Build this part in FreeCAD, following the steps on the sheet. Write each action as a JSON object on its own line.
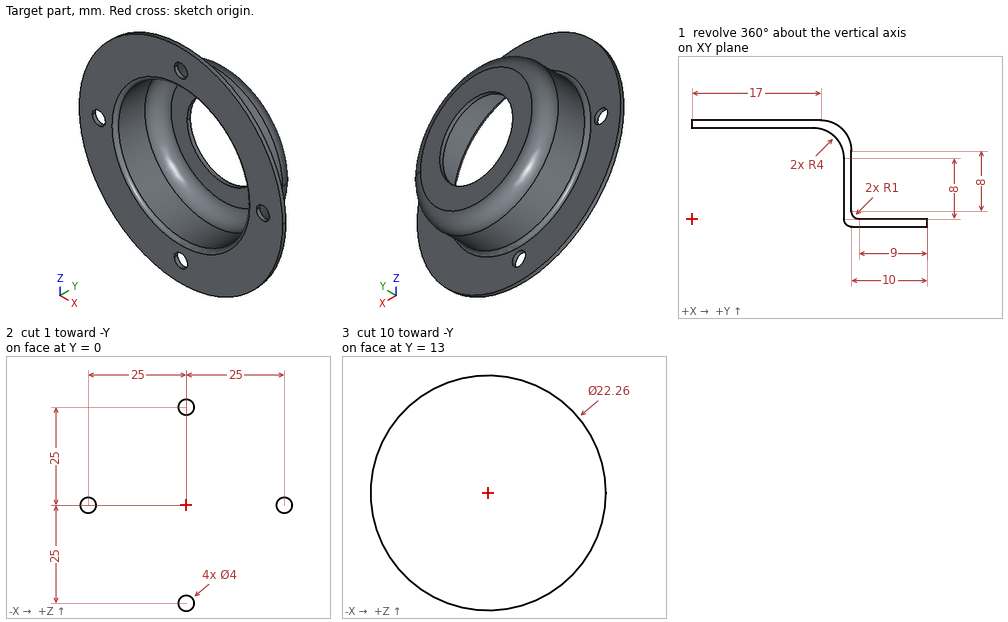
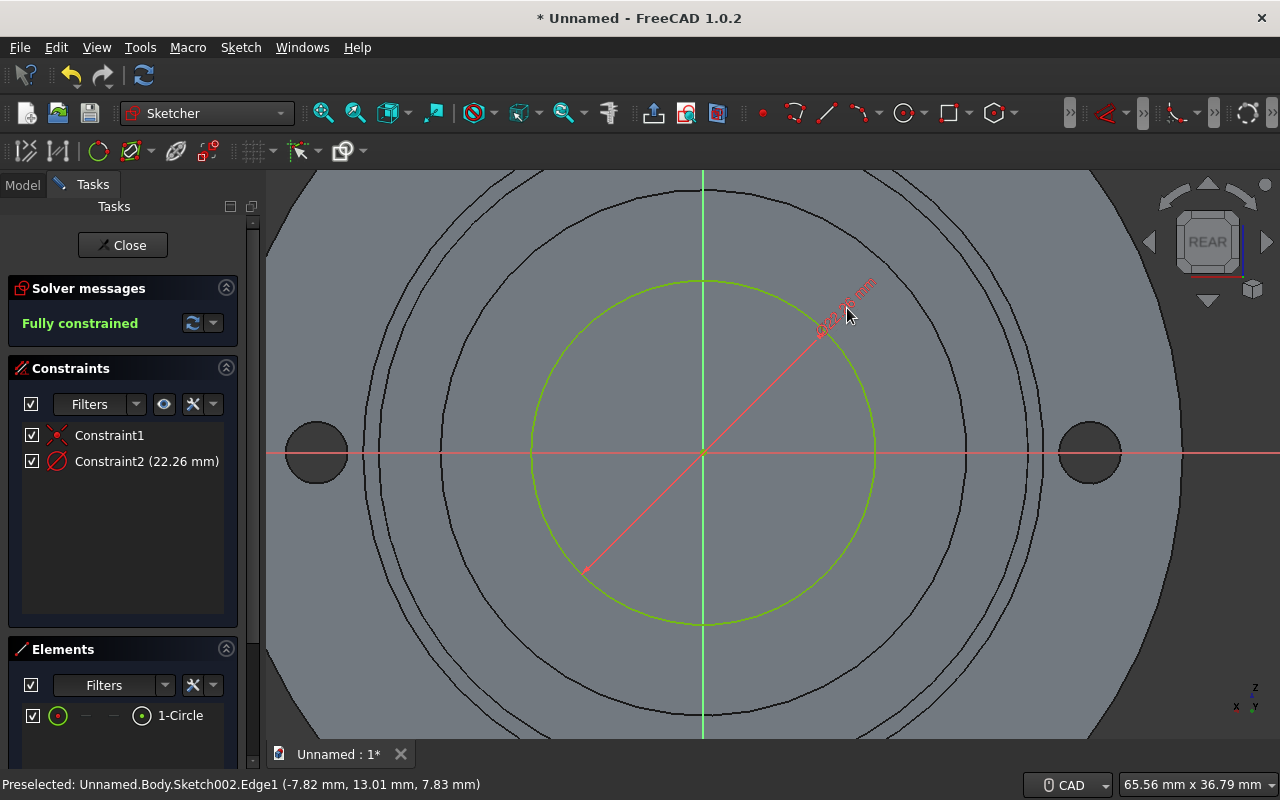
{"action": "left_click", "coordinate": [123, 245]}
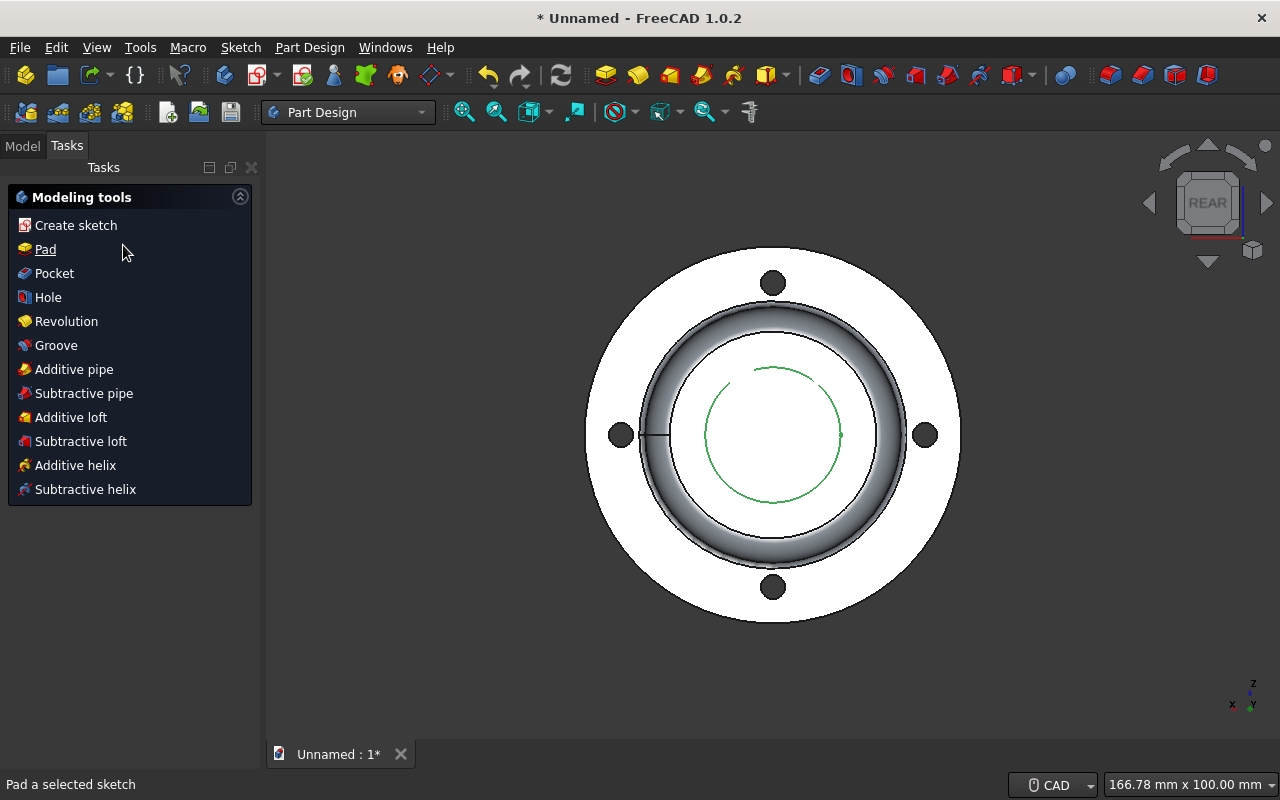
{"action": "left_click", "coordinate": [820, 76]}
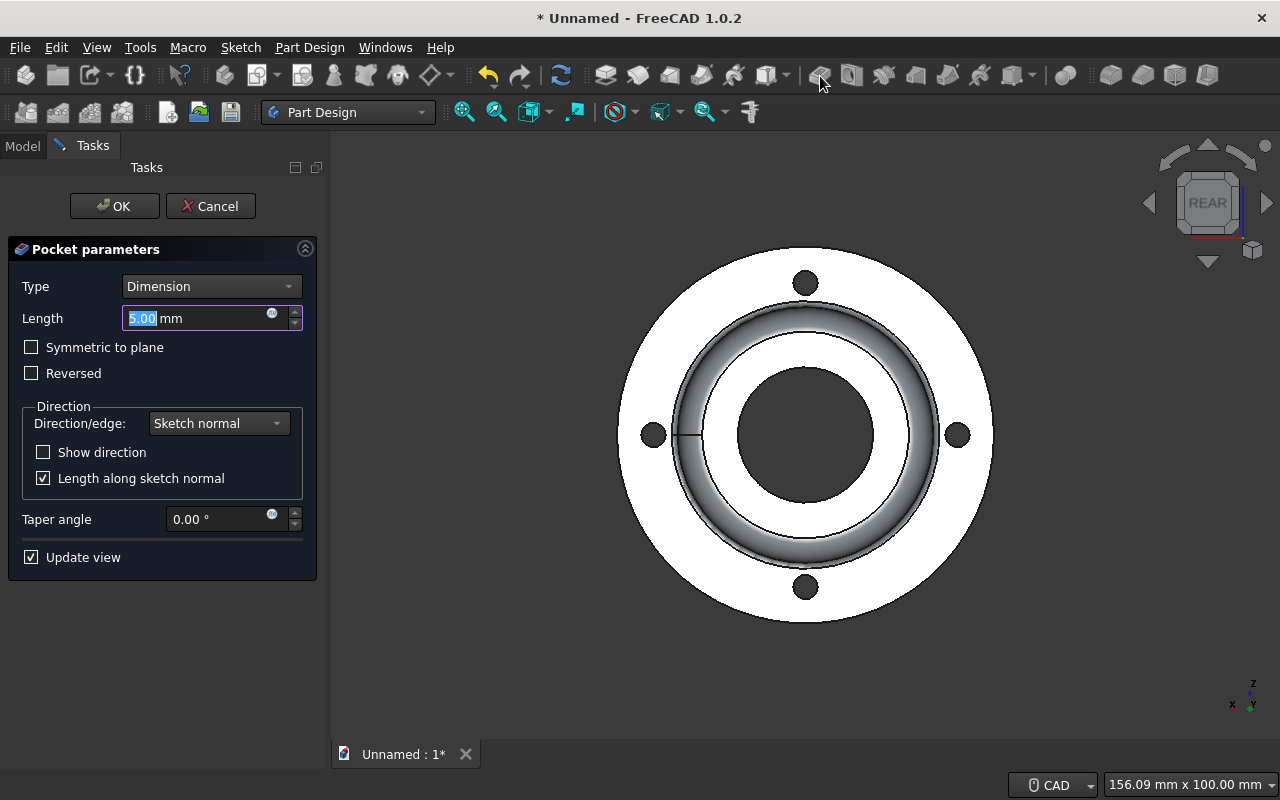
{"action": "type", "text": "10"}
{"action": "key", "text": "Tab"}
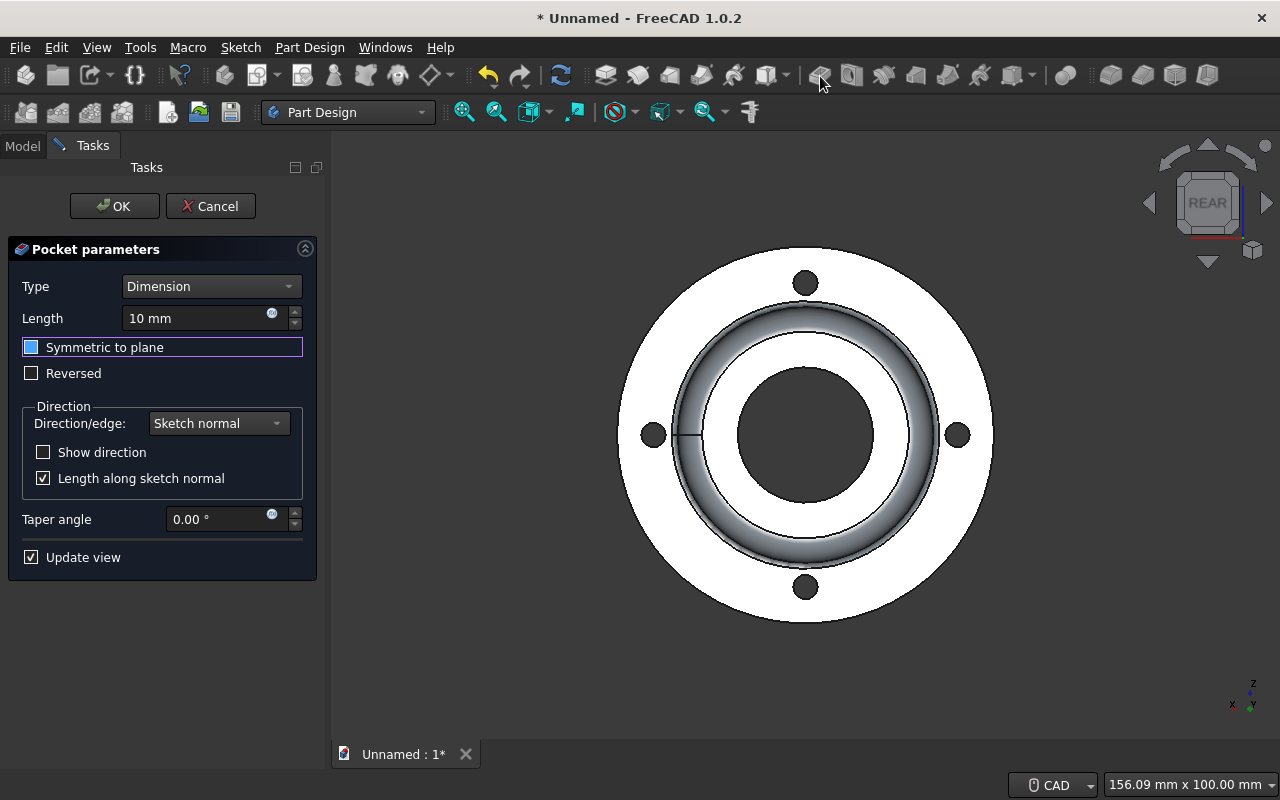
{"action": "left_click", "coordinate": [115, 206]}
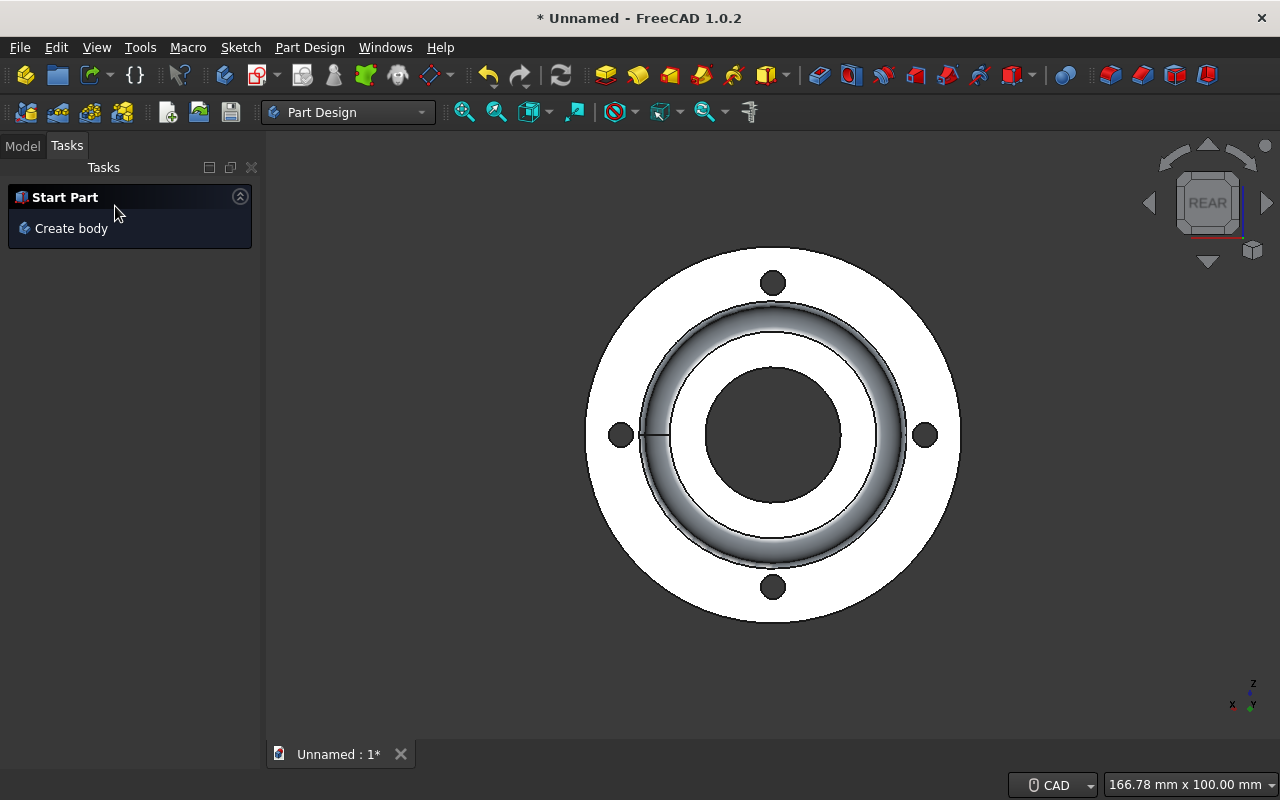
{"action": "key", "text": "0"}